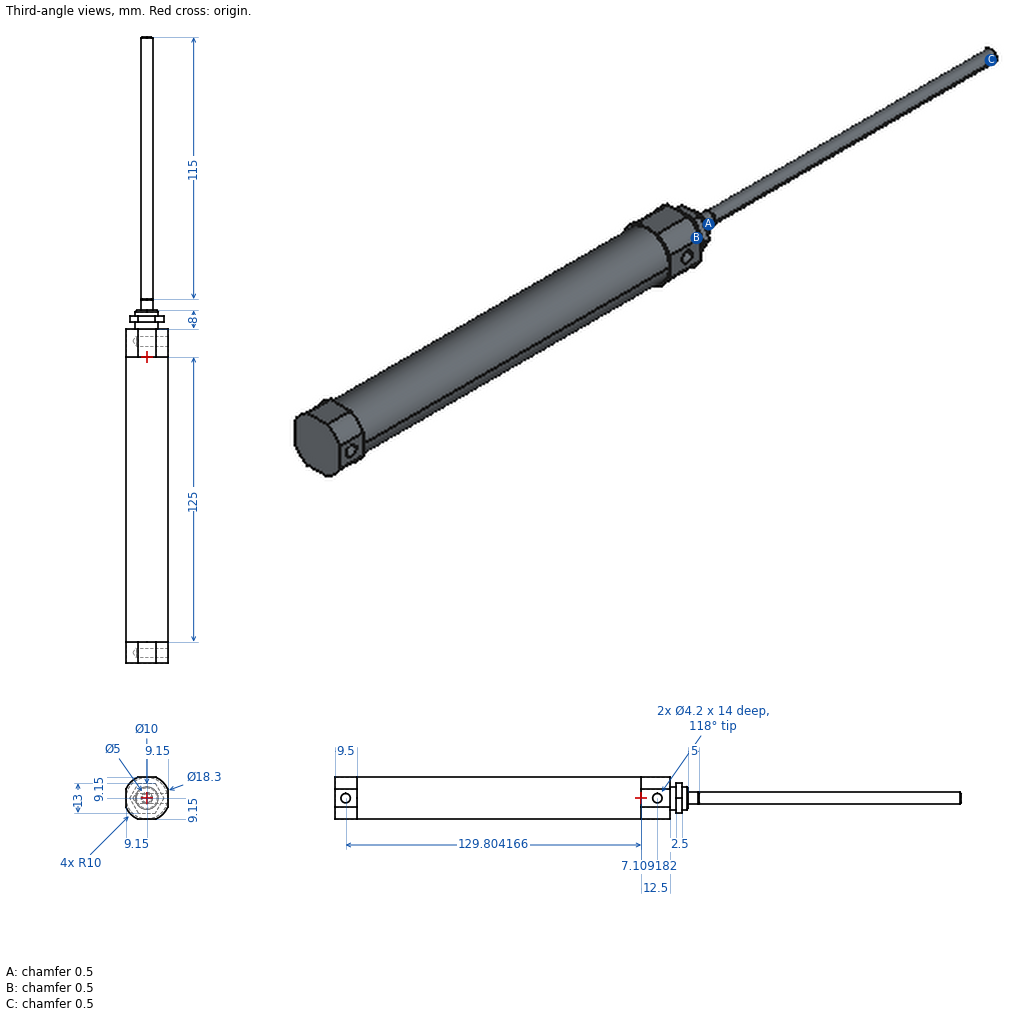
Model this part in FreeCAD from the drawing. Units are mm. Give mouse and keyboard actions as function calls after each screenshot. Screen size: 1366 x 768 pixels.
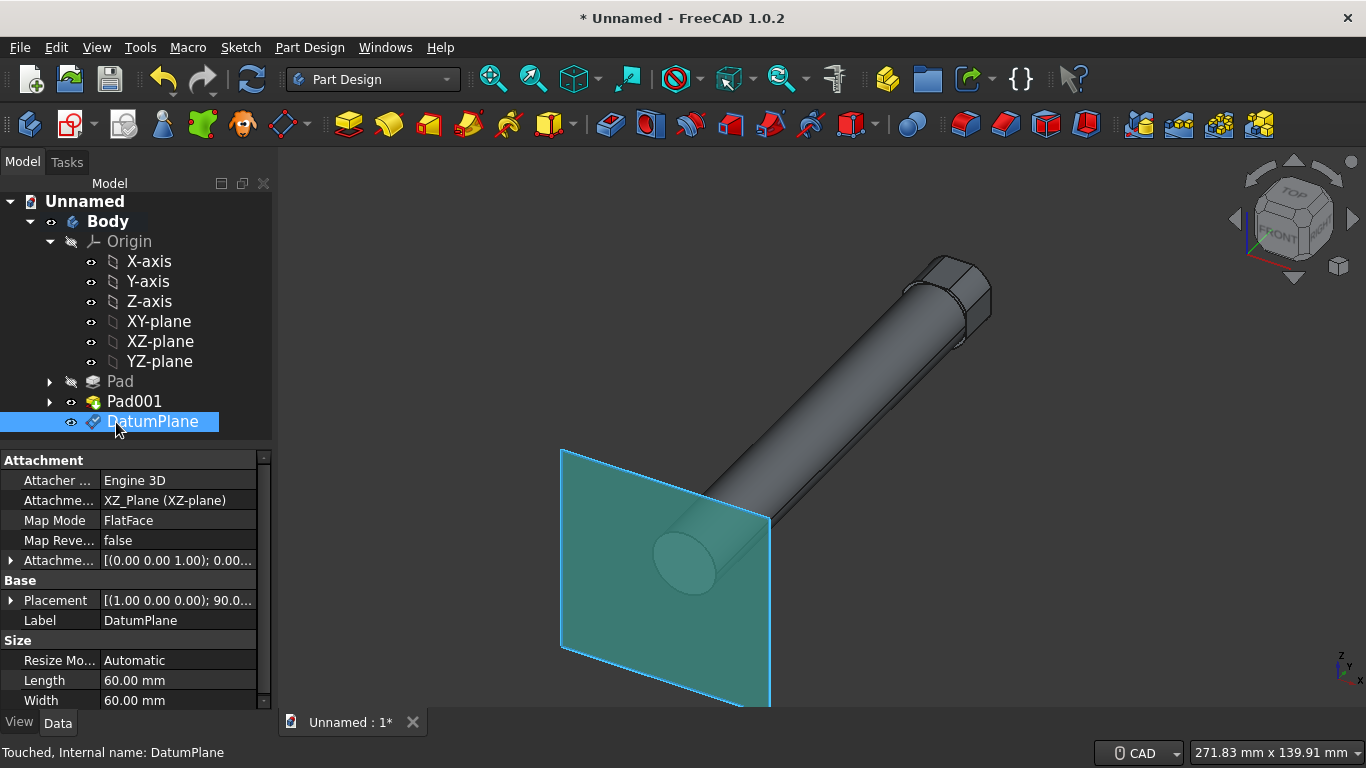
click(70, 124)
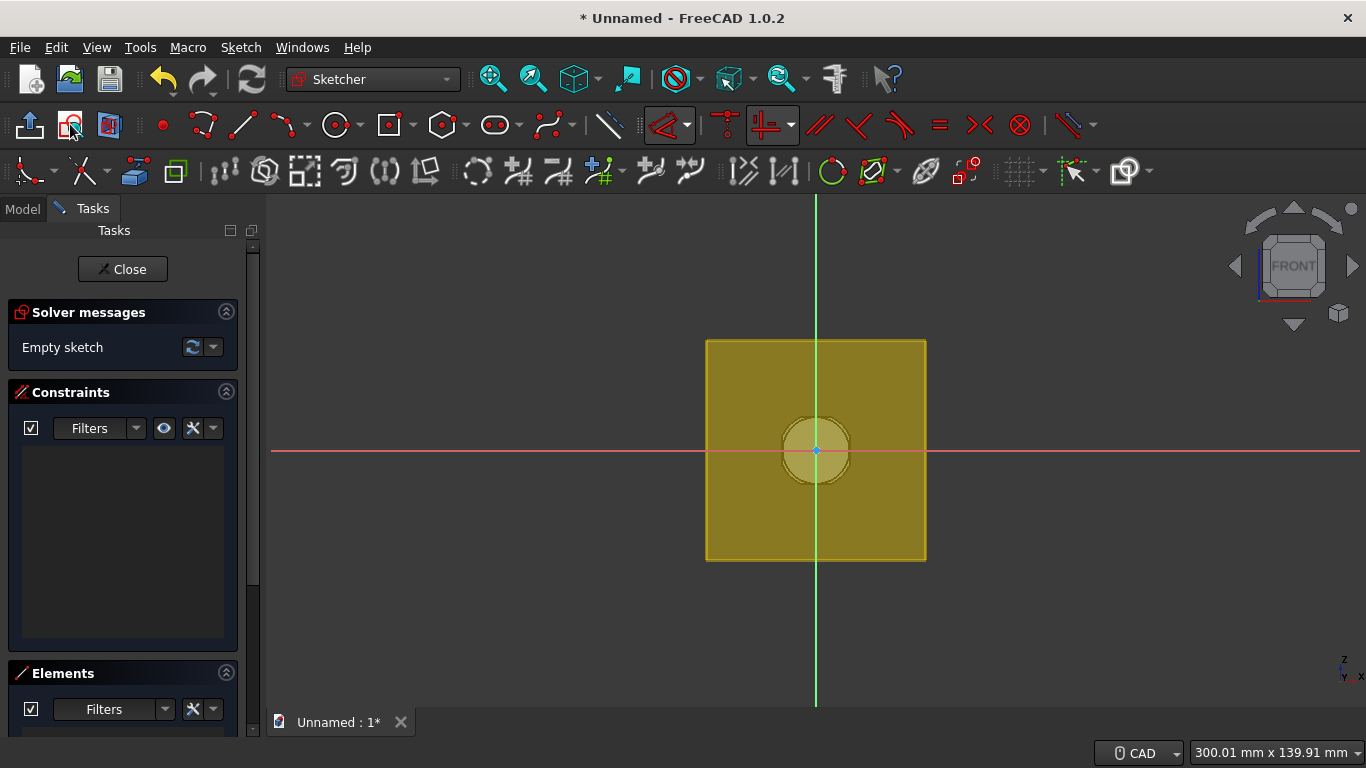
scroll(833, 450, up, 8)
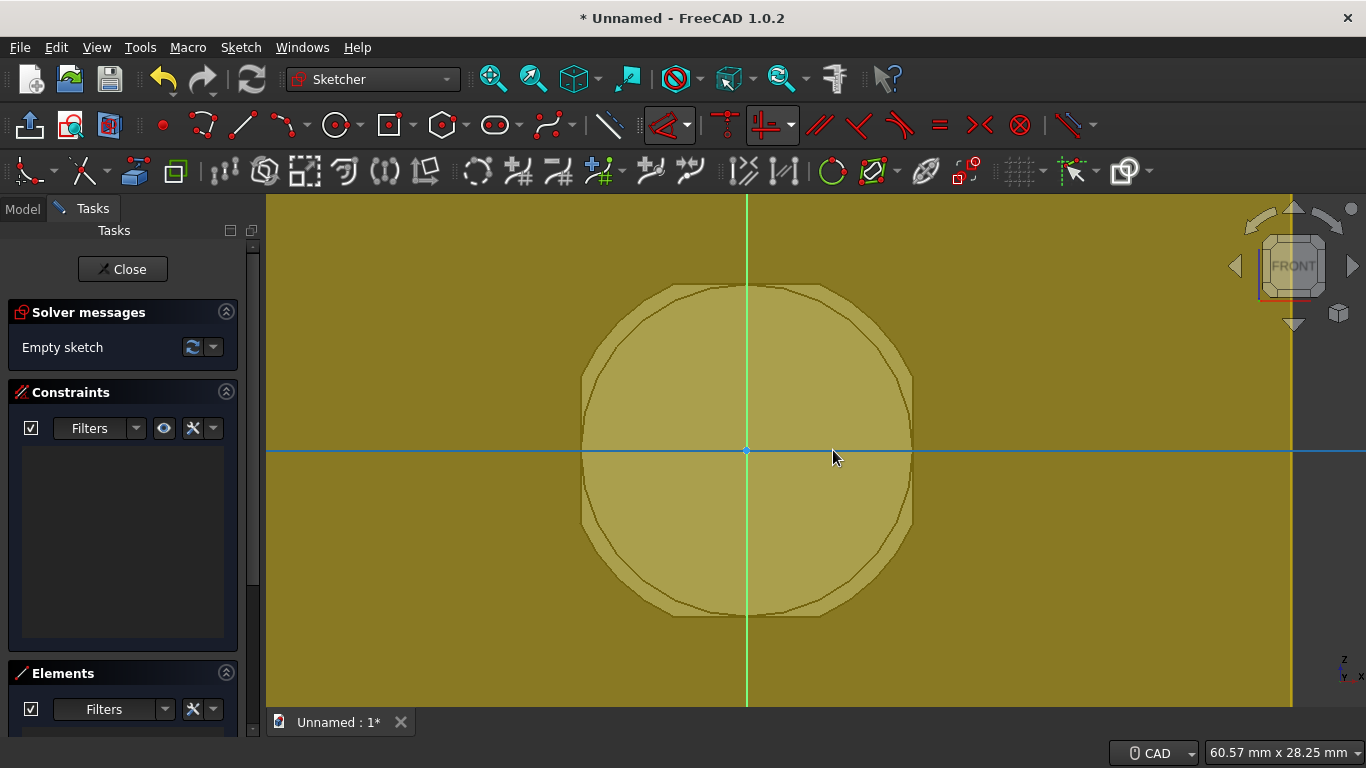
key(g)
key(l)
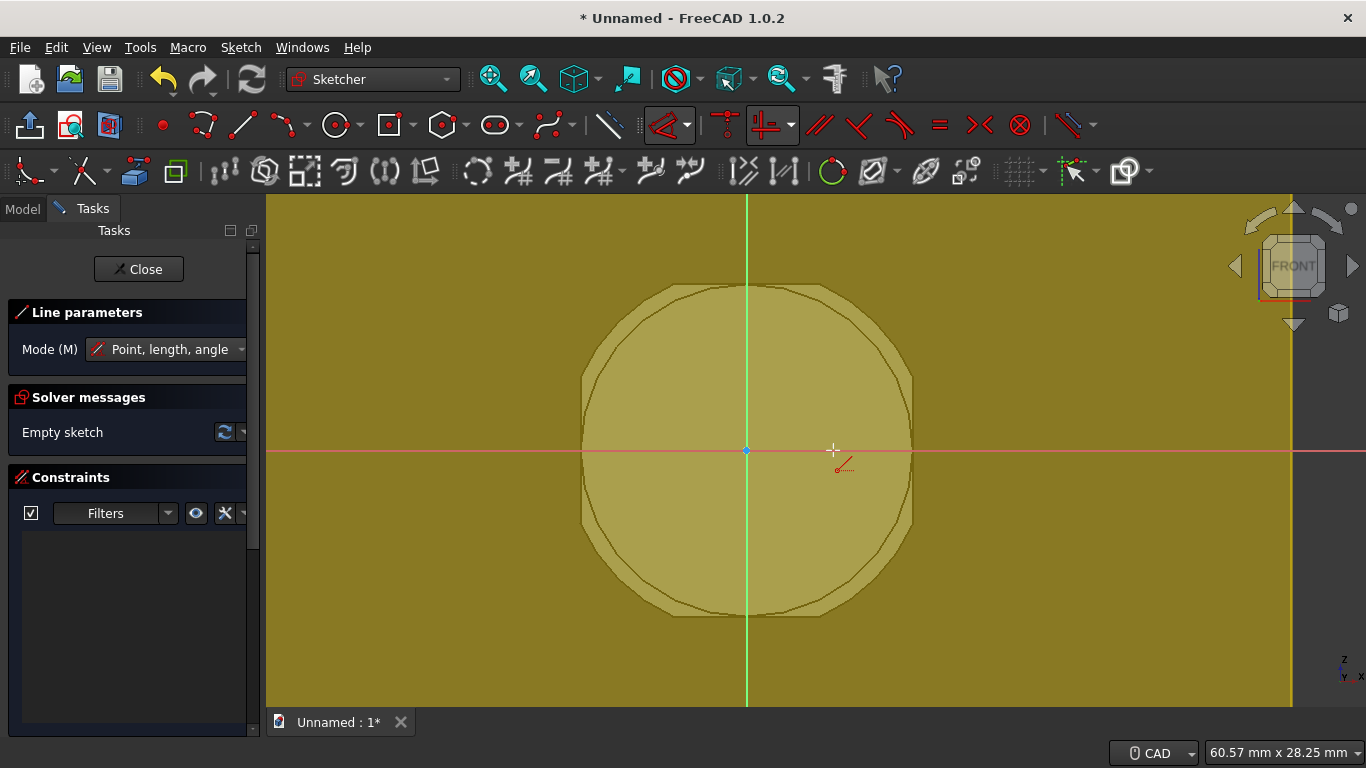
click(820, 284)
click(673, 284)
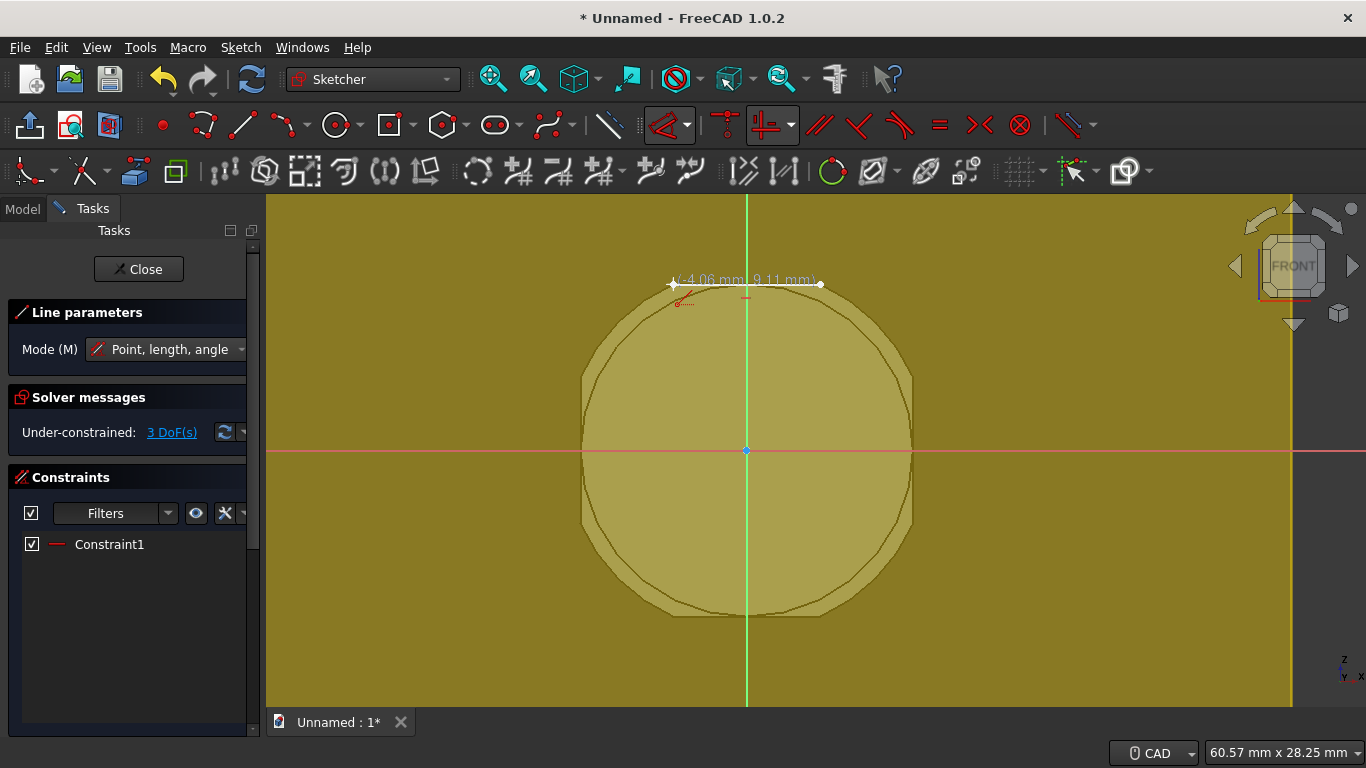
click(581, 377)
click(581, 524)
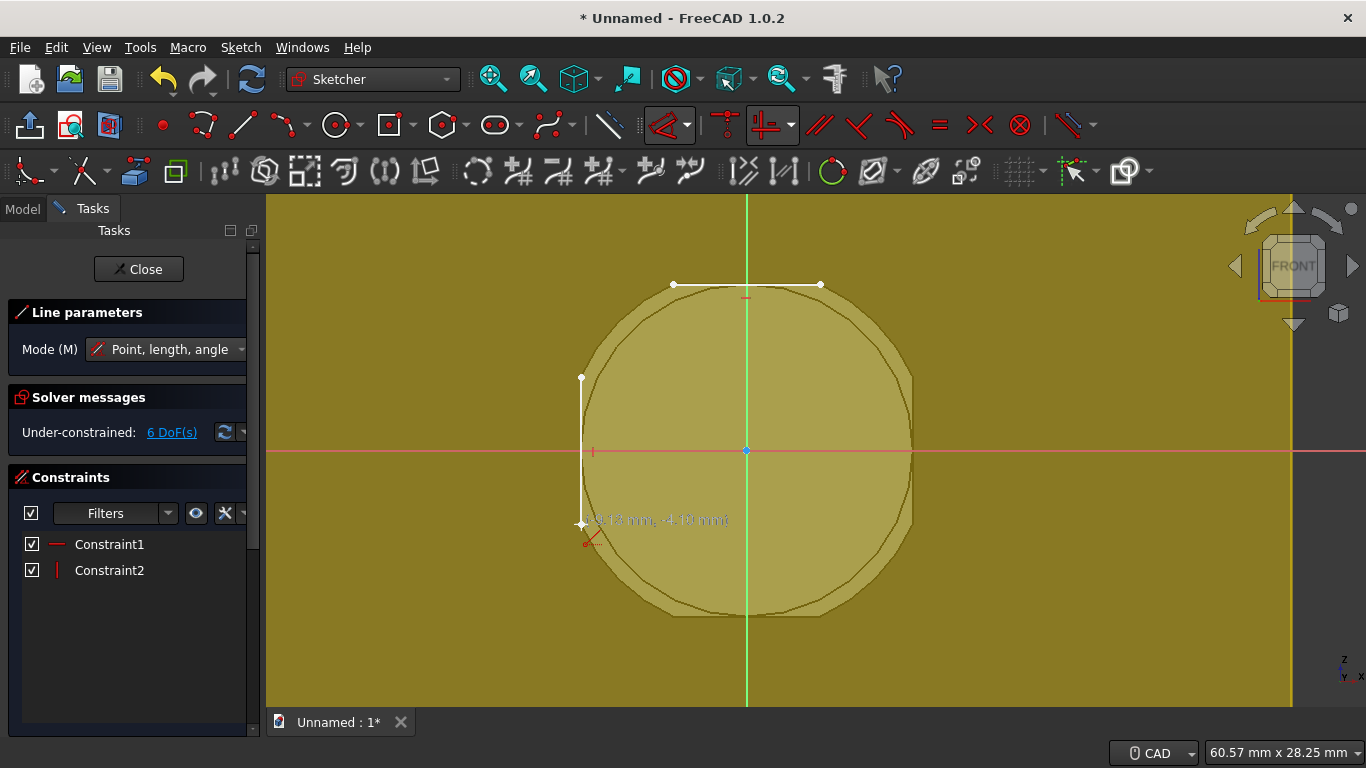
click(673, 617)
click(820, 617)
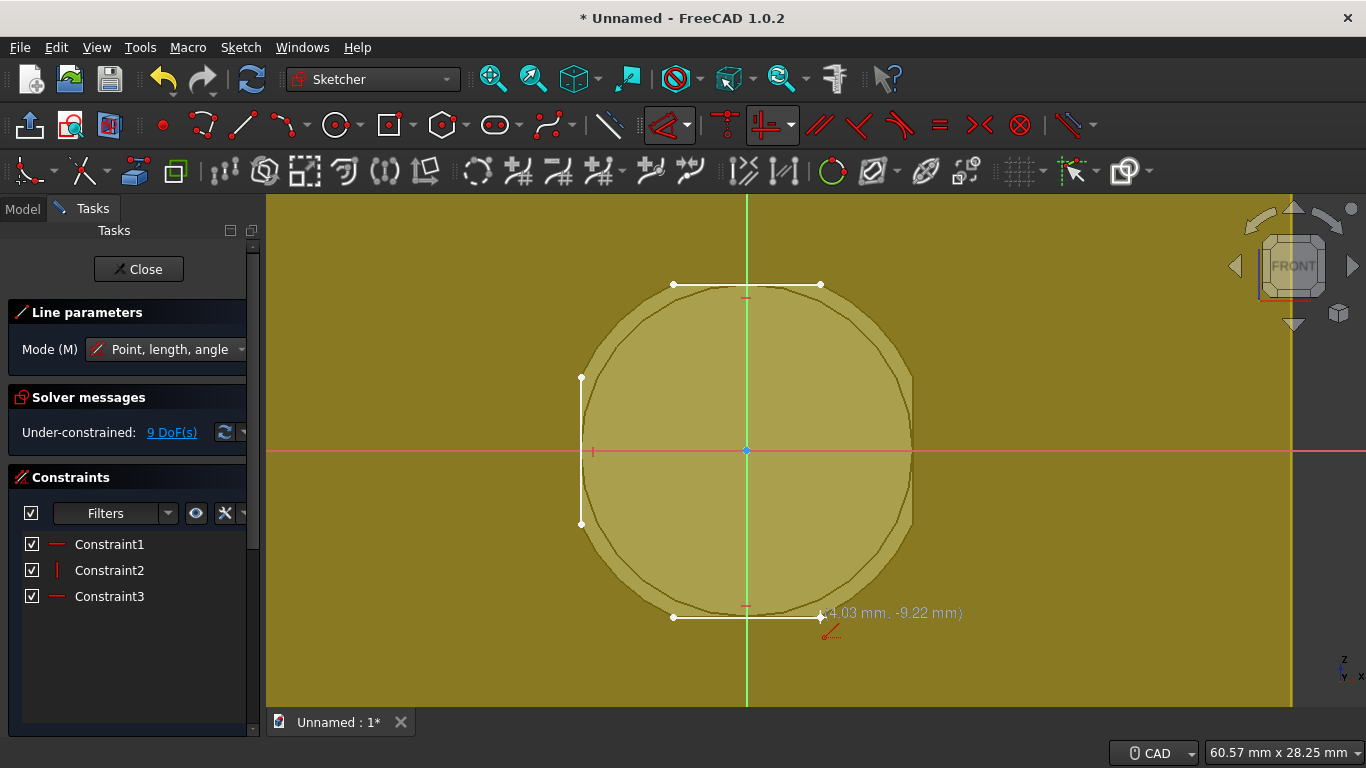
click(913, 524)
click(913, 377)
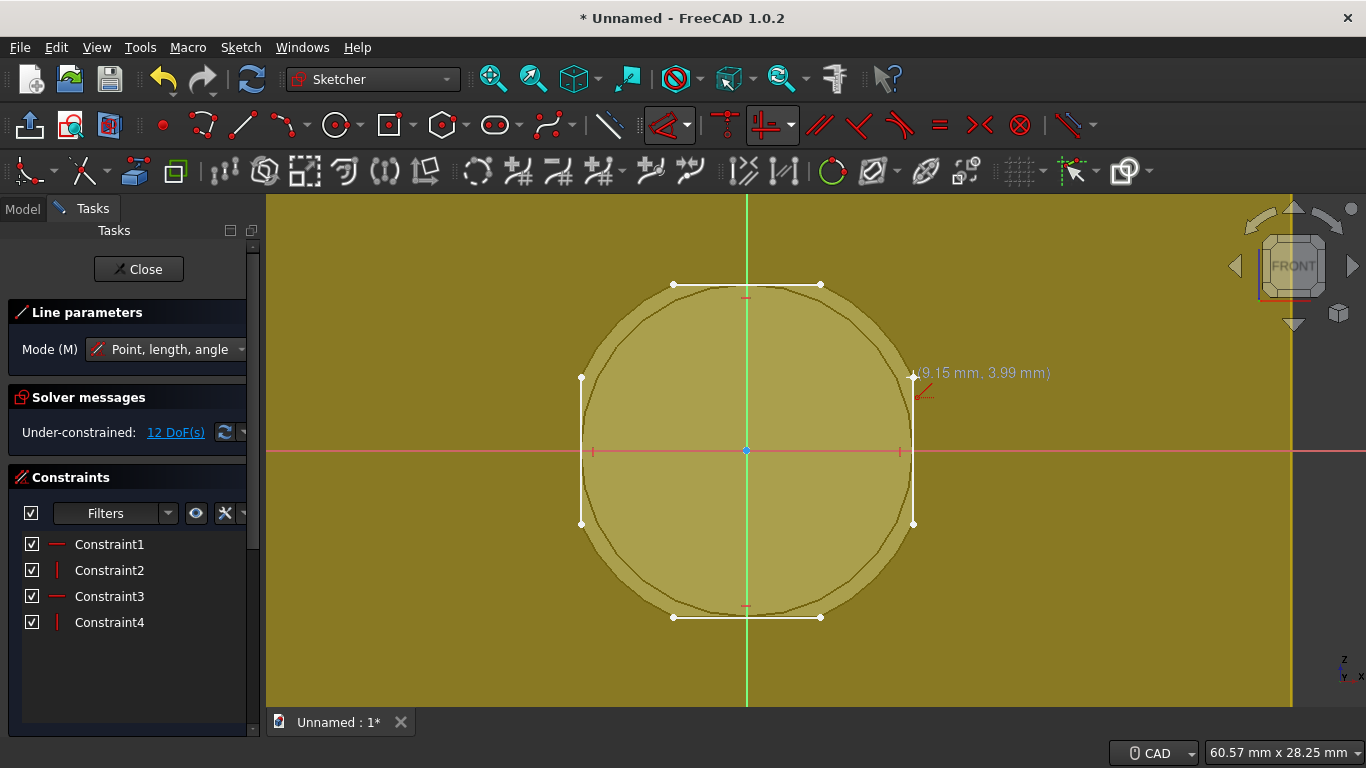
click(284, 126)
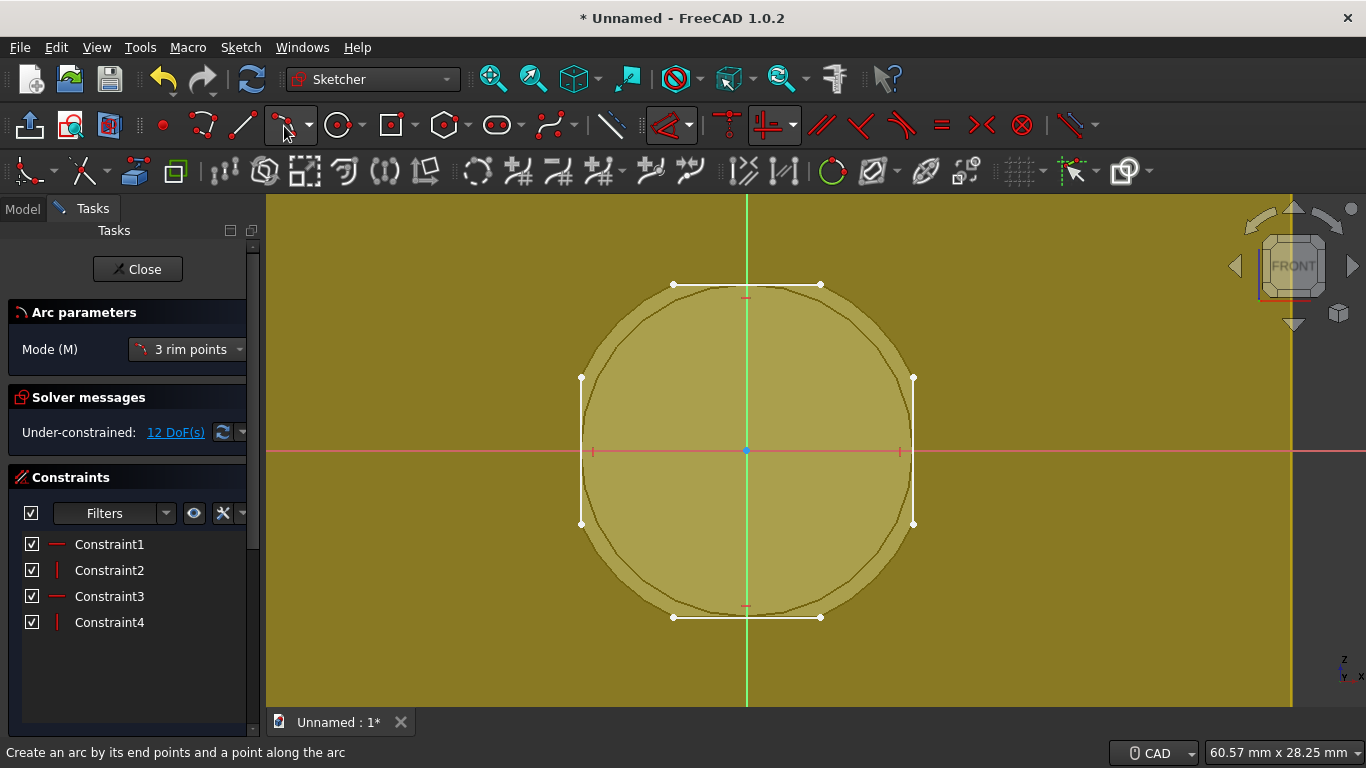
click(673, 285)
click(581, 378)